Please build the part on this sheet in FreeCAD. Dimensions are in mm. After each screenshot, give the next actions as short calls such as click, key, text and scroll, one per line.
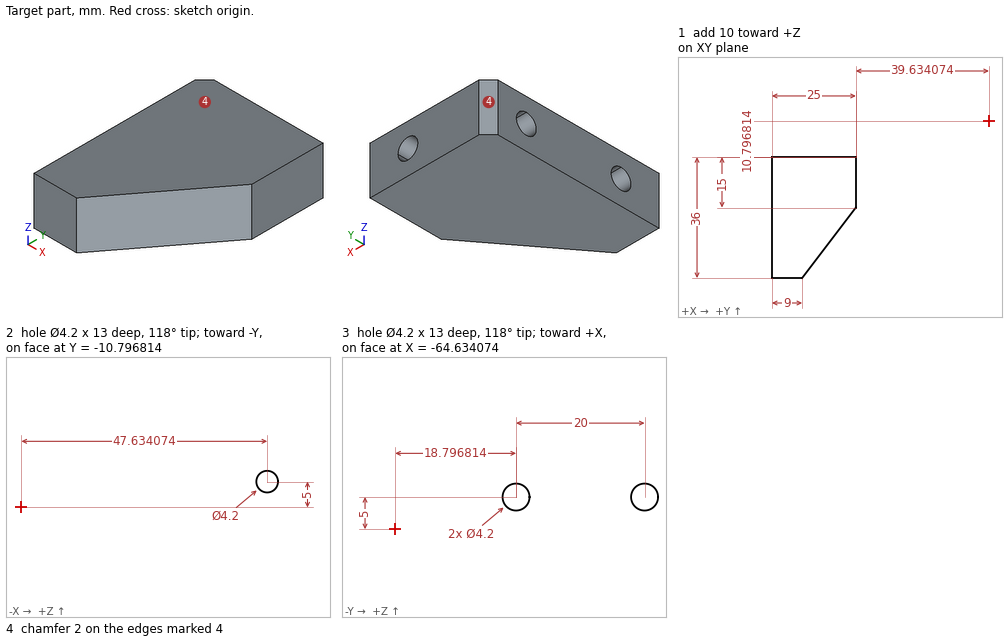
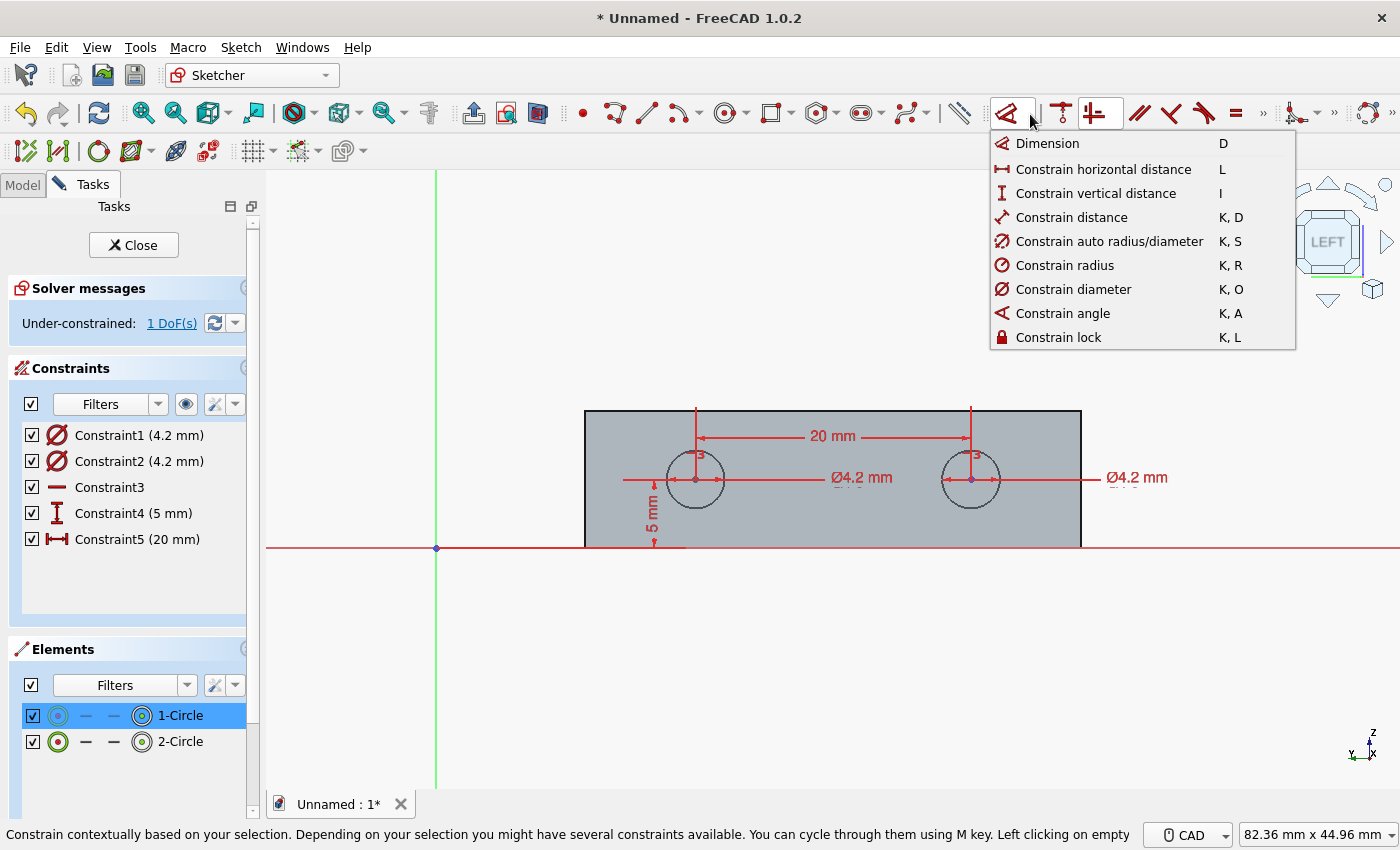
click(1143, 169)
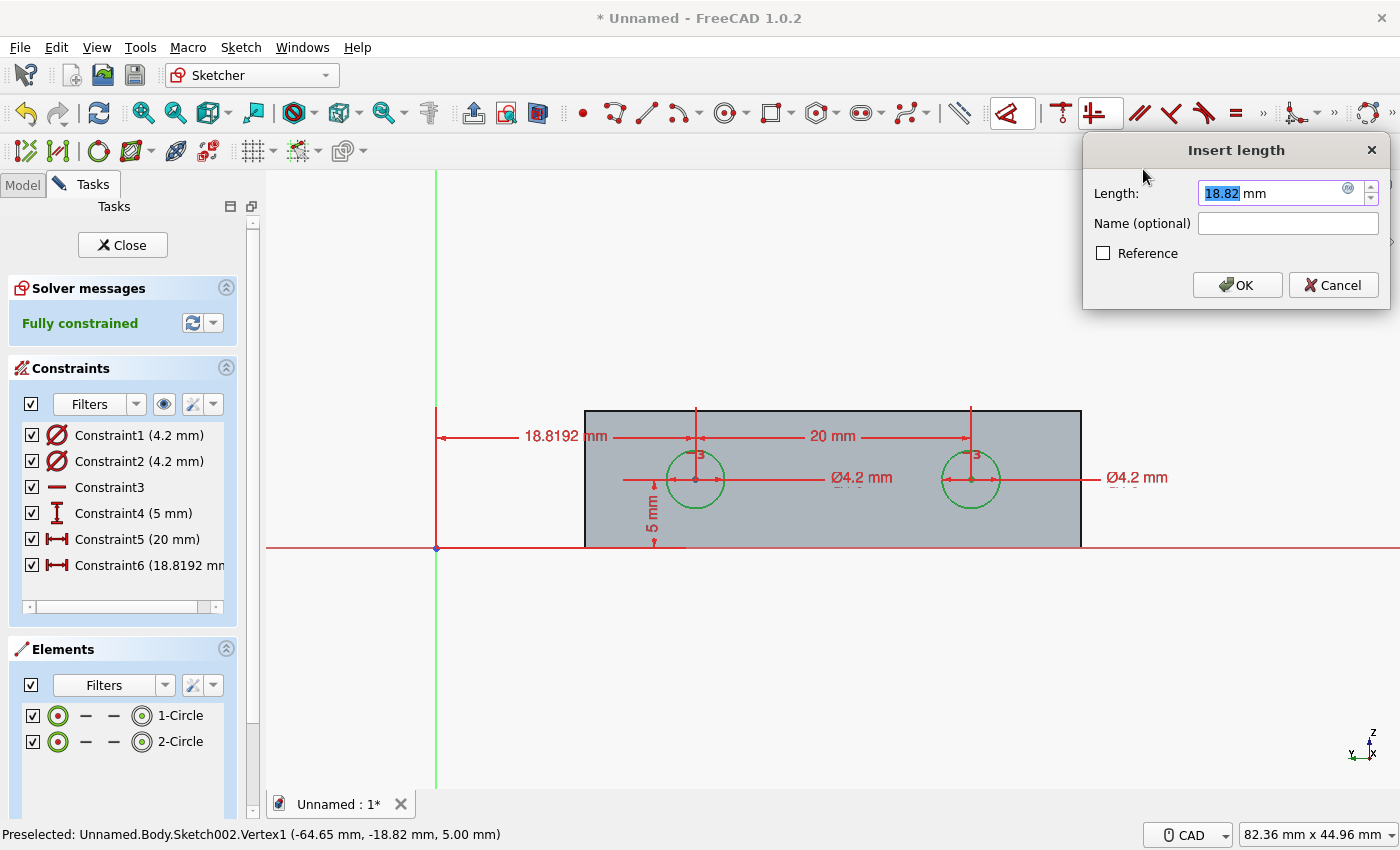
text(18.796814)
key(Return)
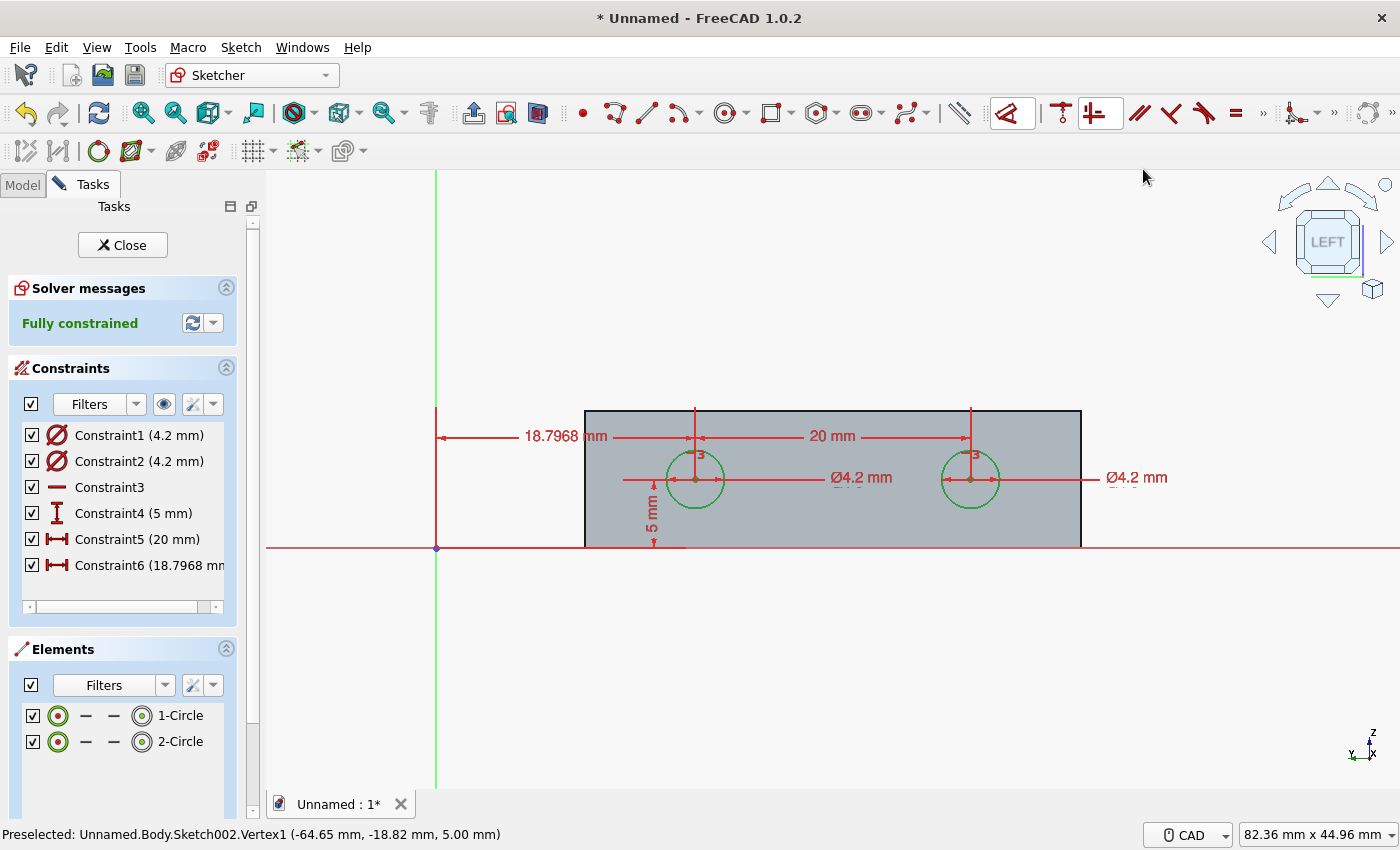
click(123, 245)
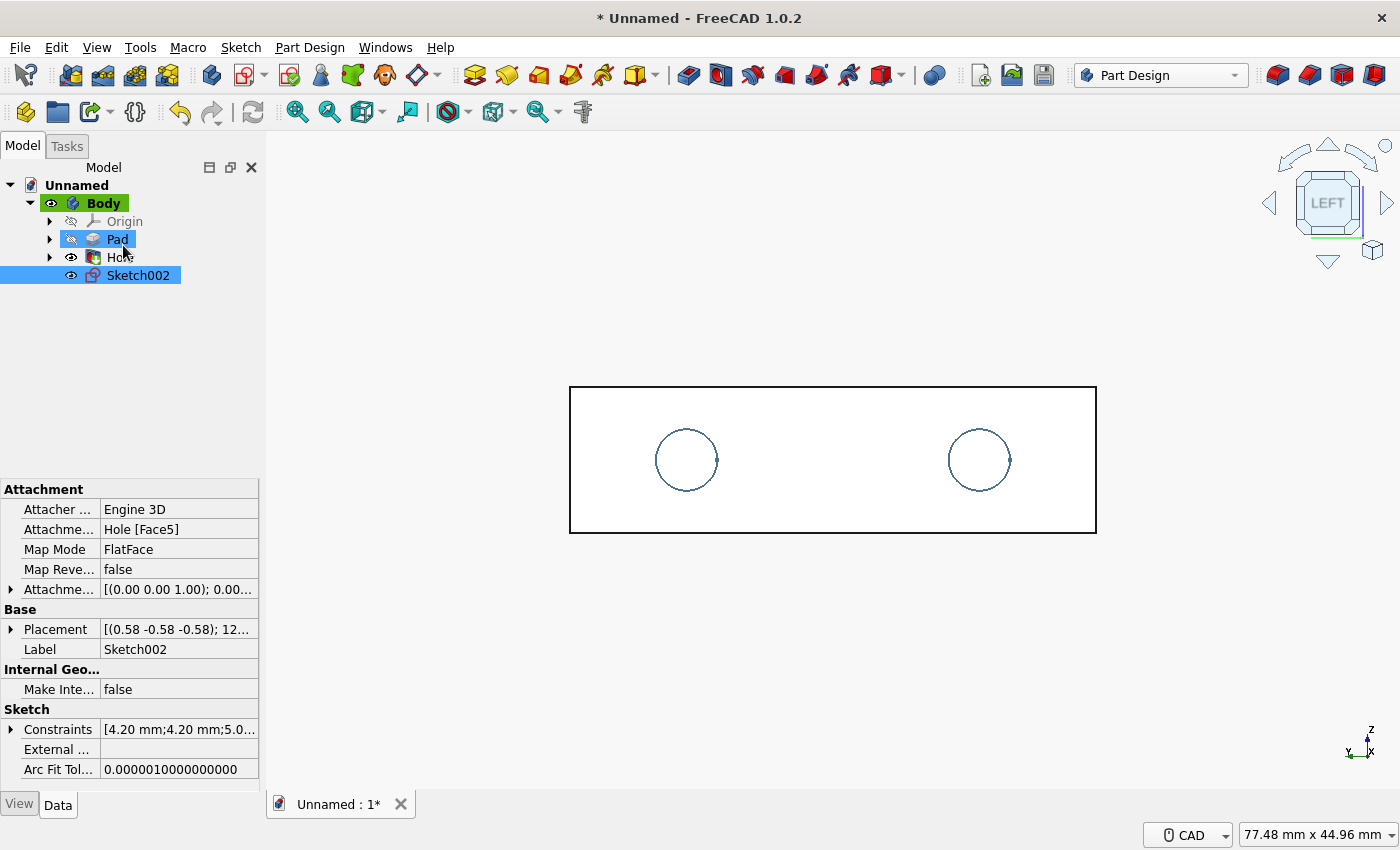
click(722, 76)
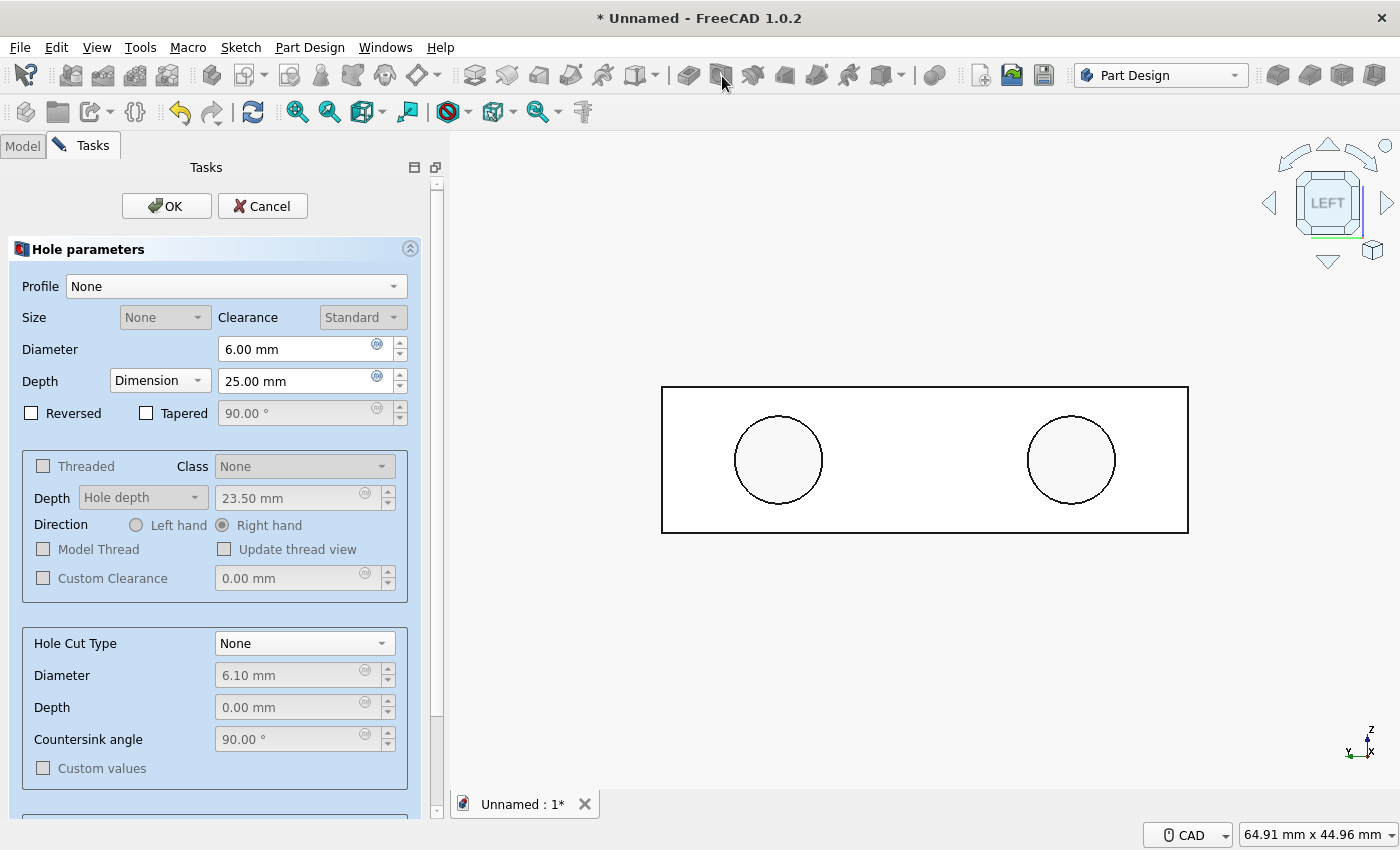
triple_click(305, 349)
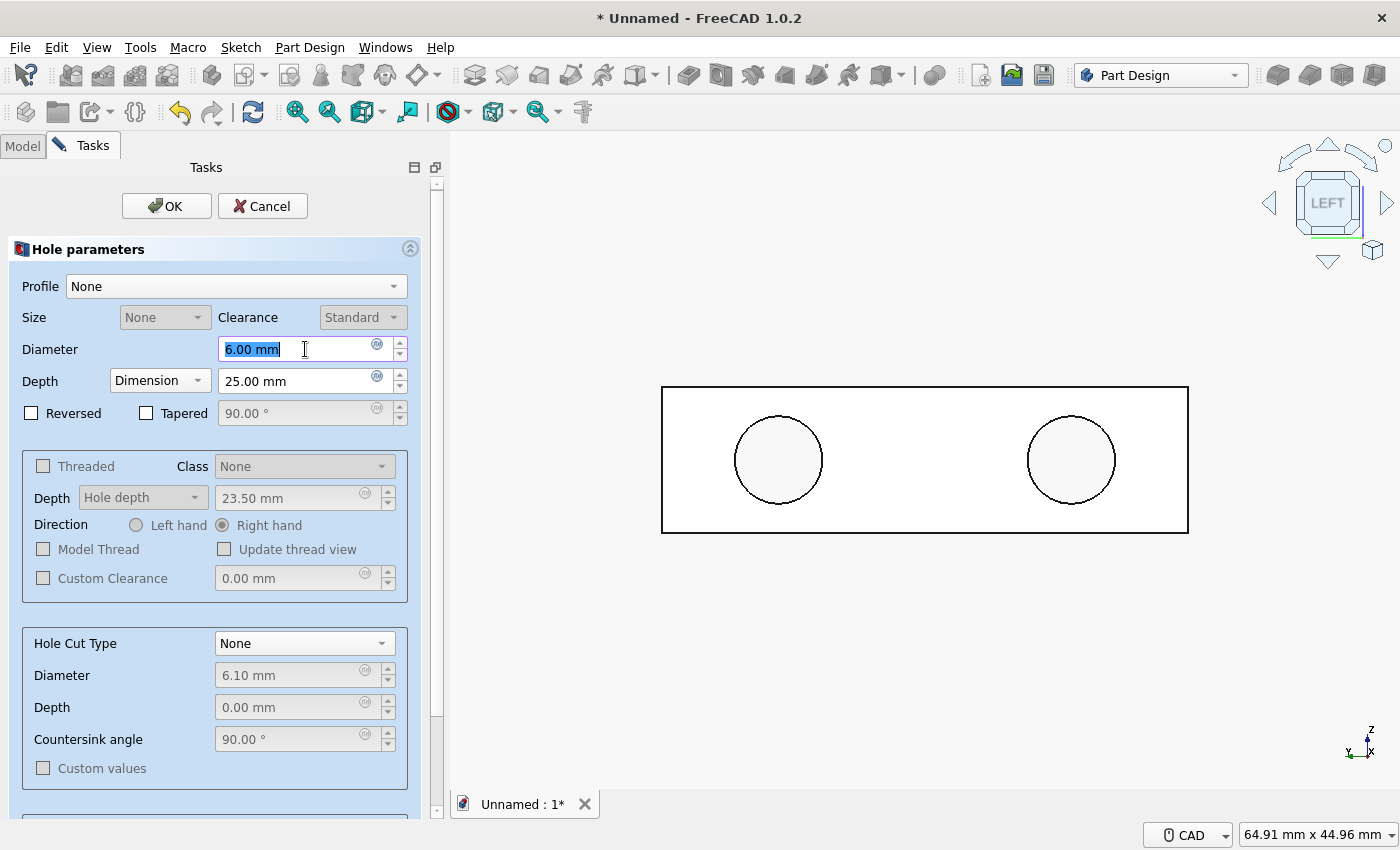
text(4.2)
key(Tab)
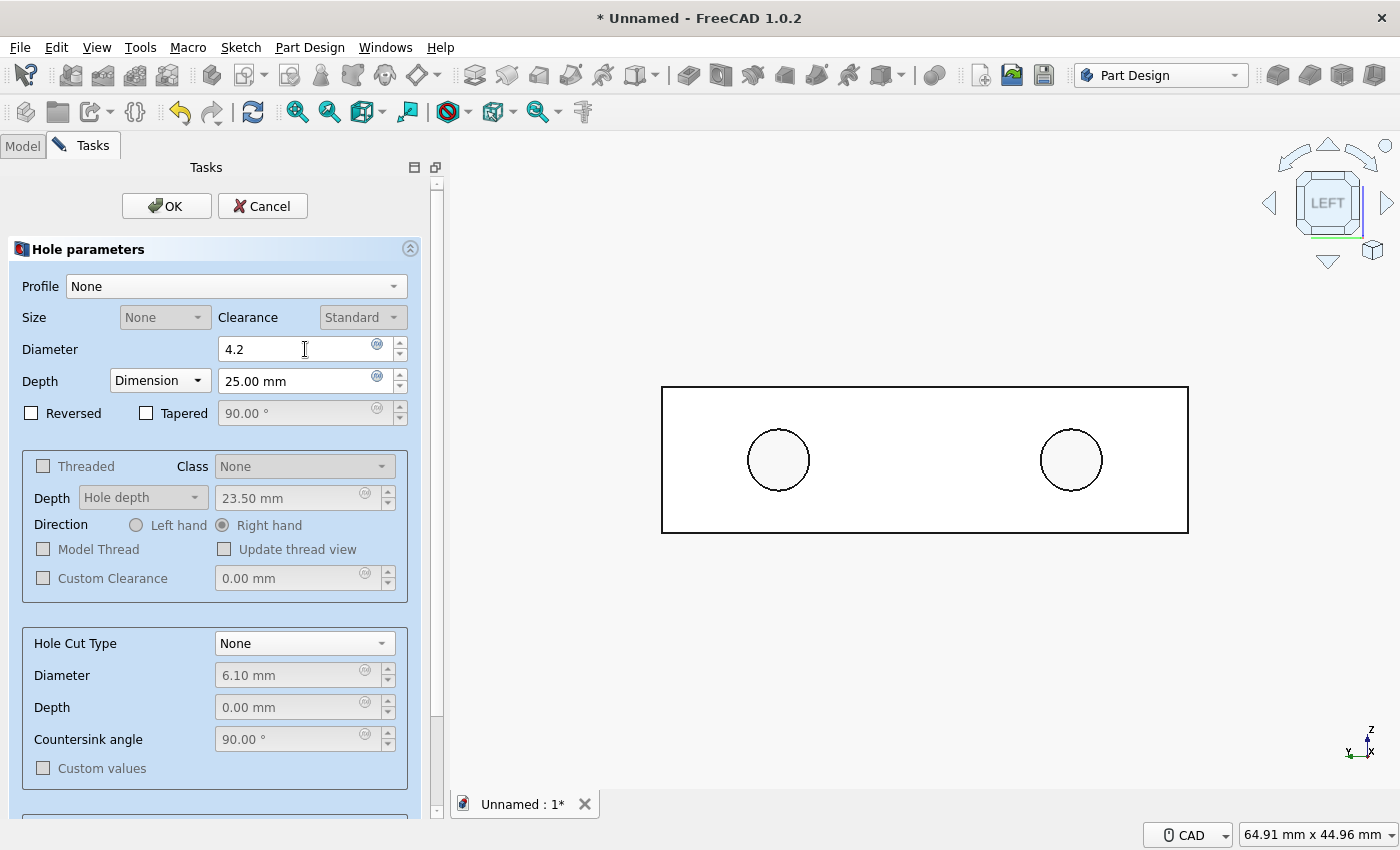
triple_click(305, 381)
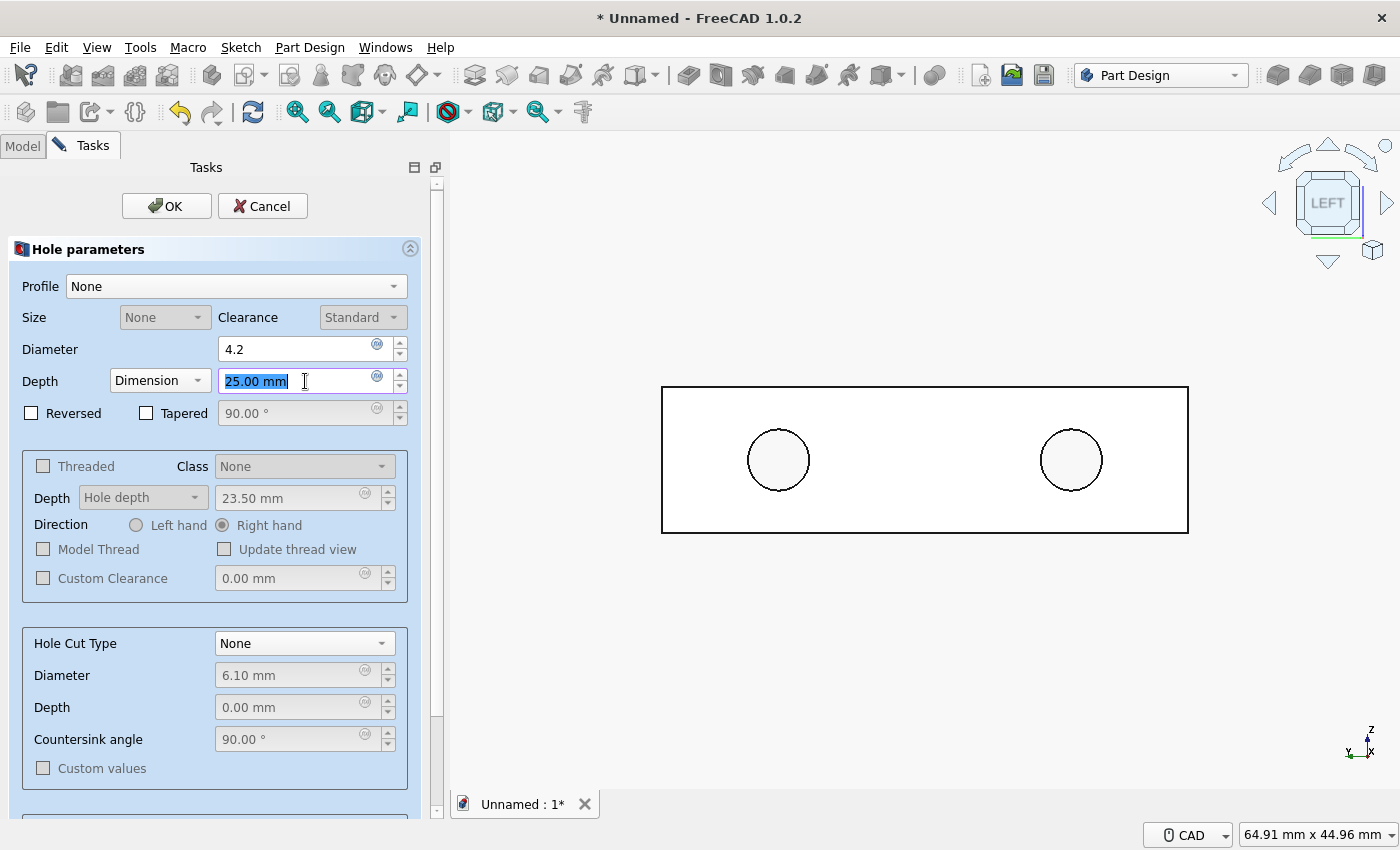
text(13)
key(Tab)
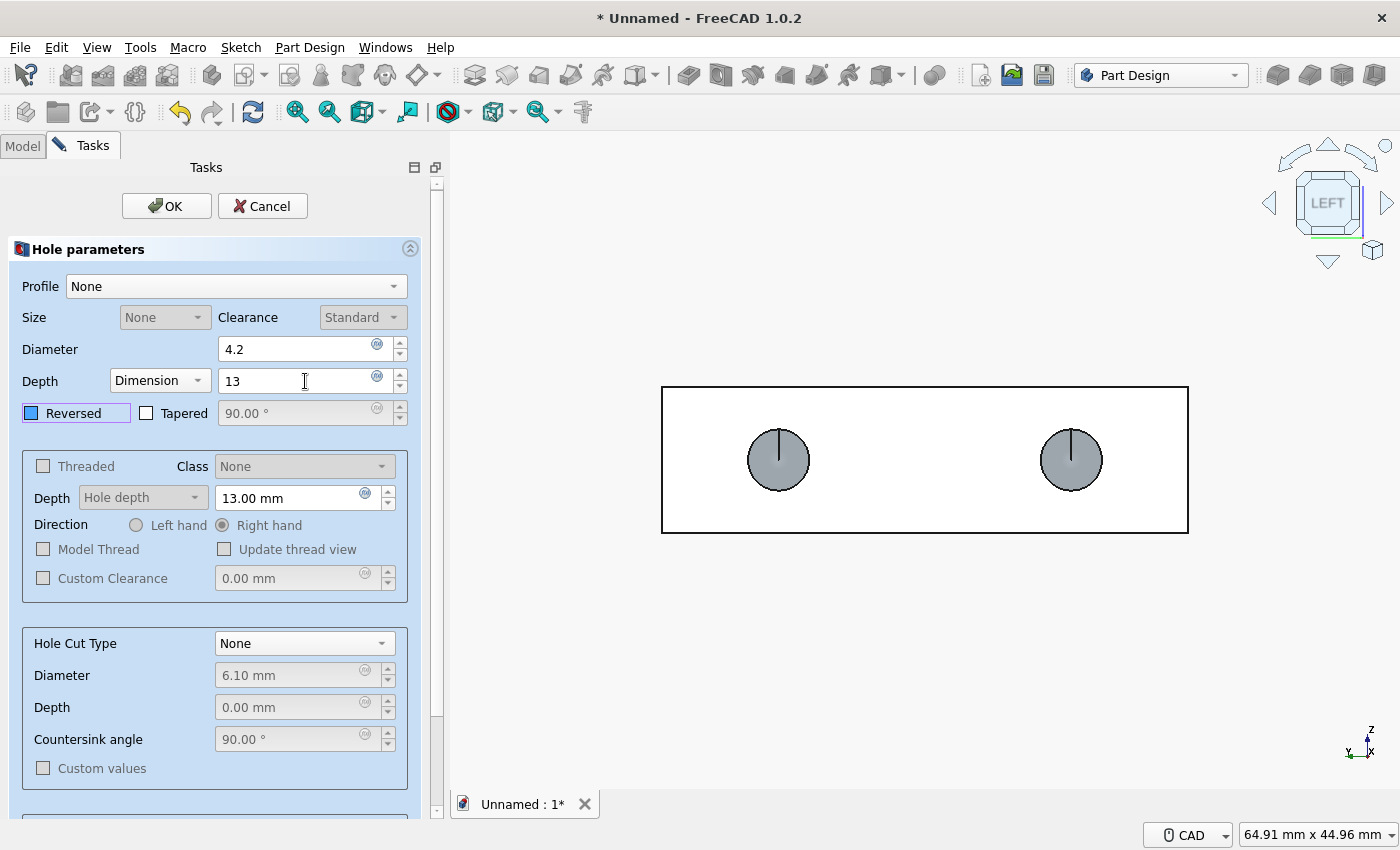
click(167, 206)